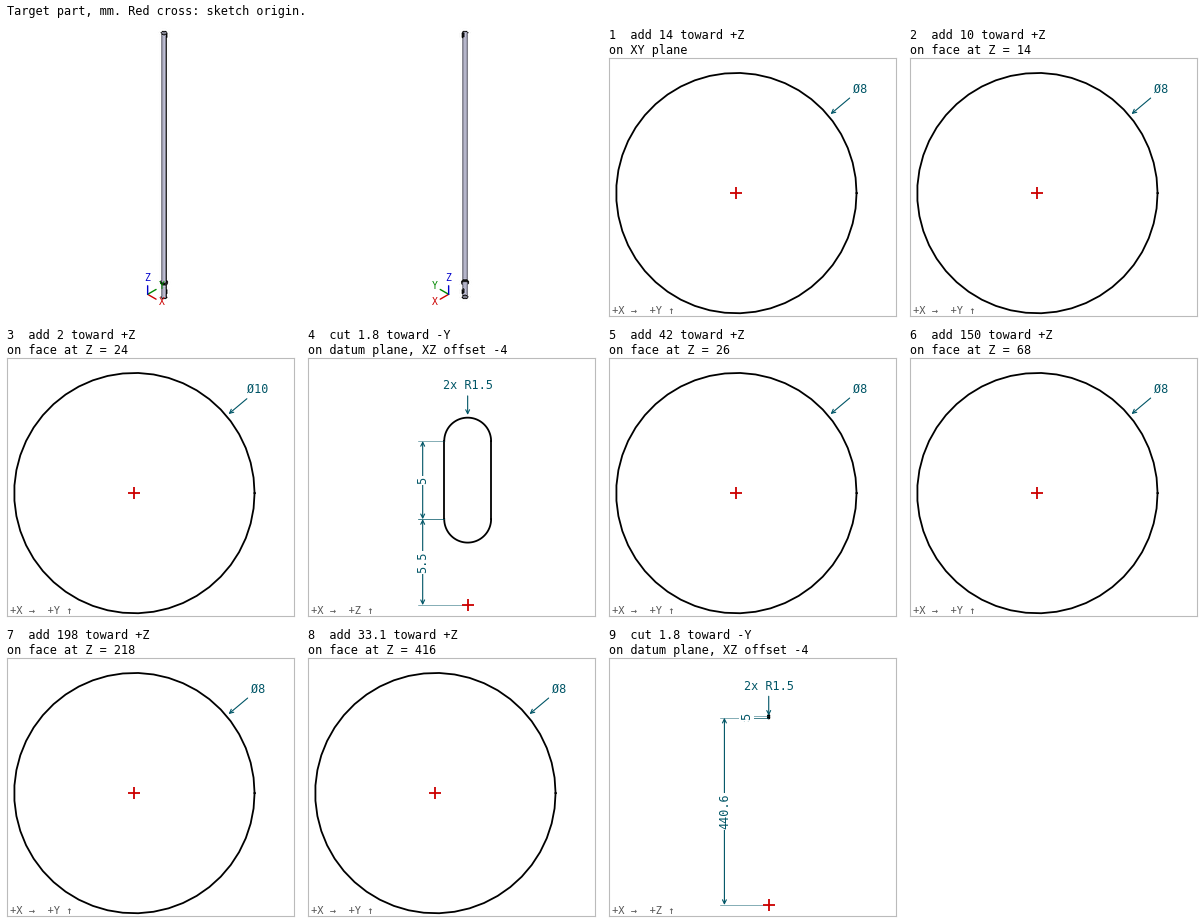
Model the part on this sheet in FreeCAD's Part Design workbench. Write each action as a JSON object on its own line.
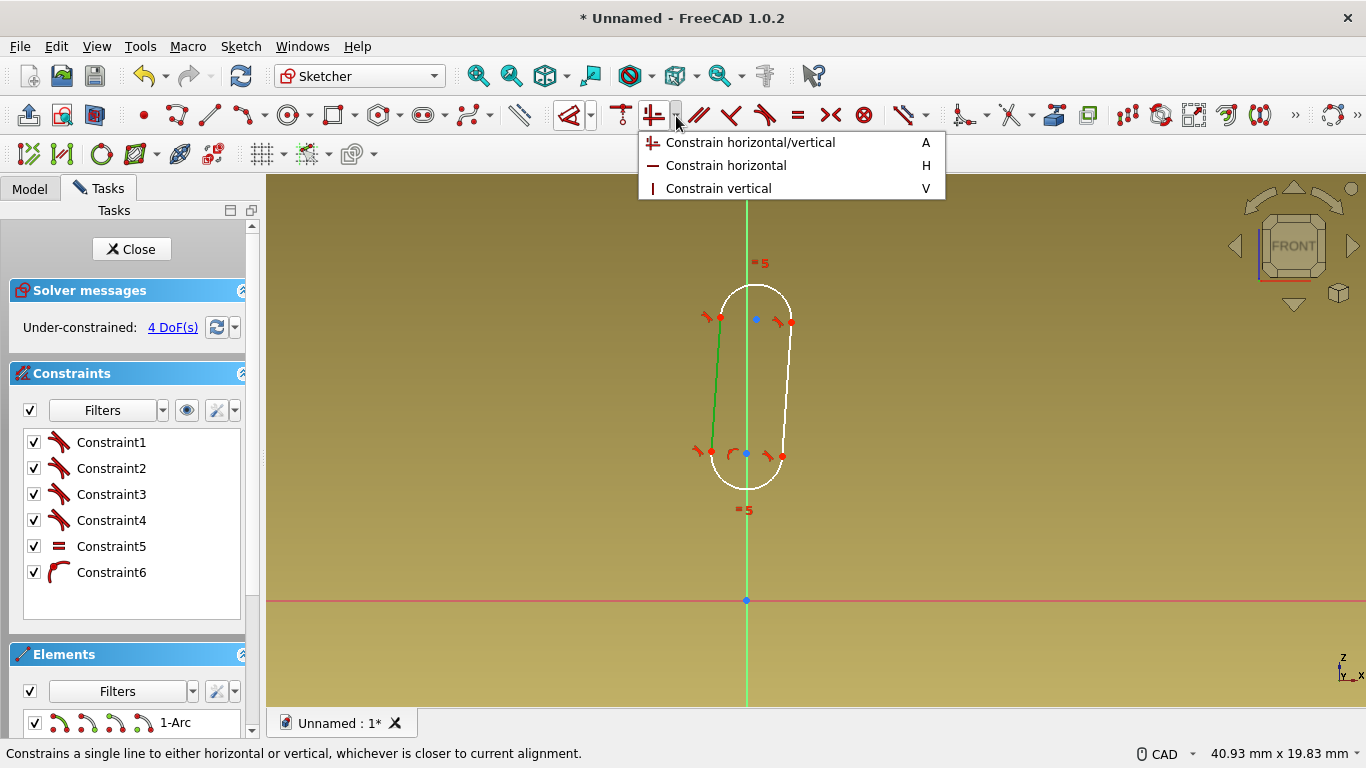
{"action": "left_click", "coordinate": [792, 188]}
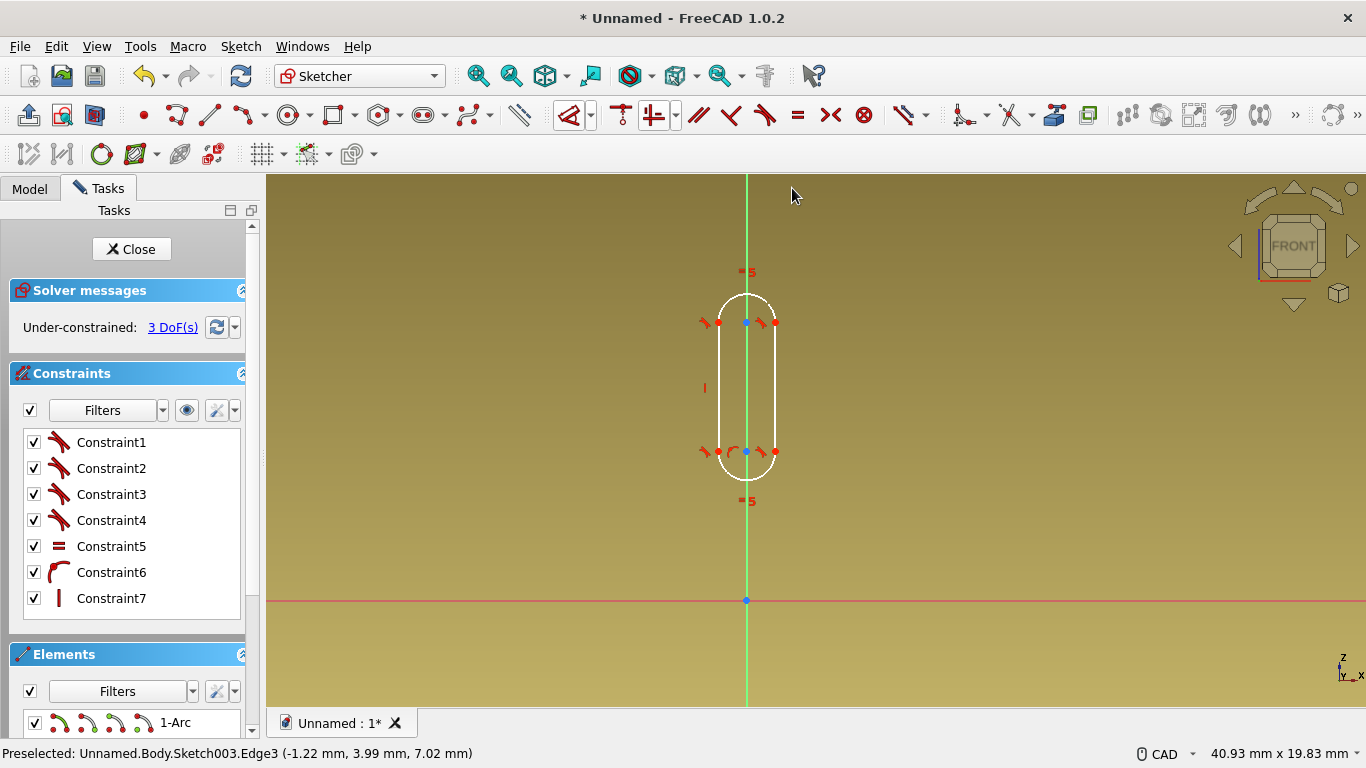
{"action": "left_click", "coordinate": [730, 475]}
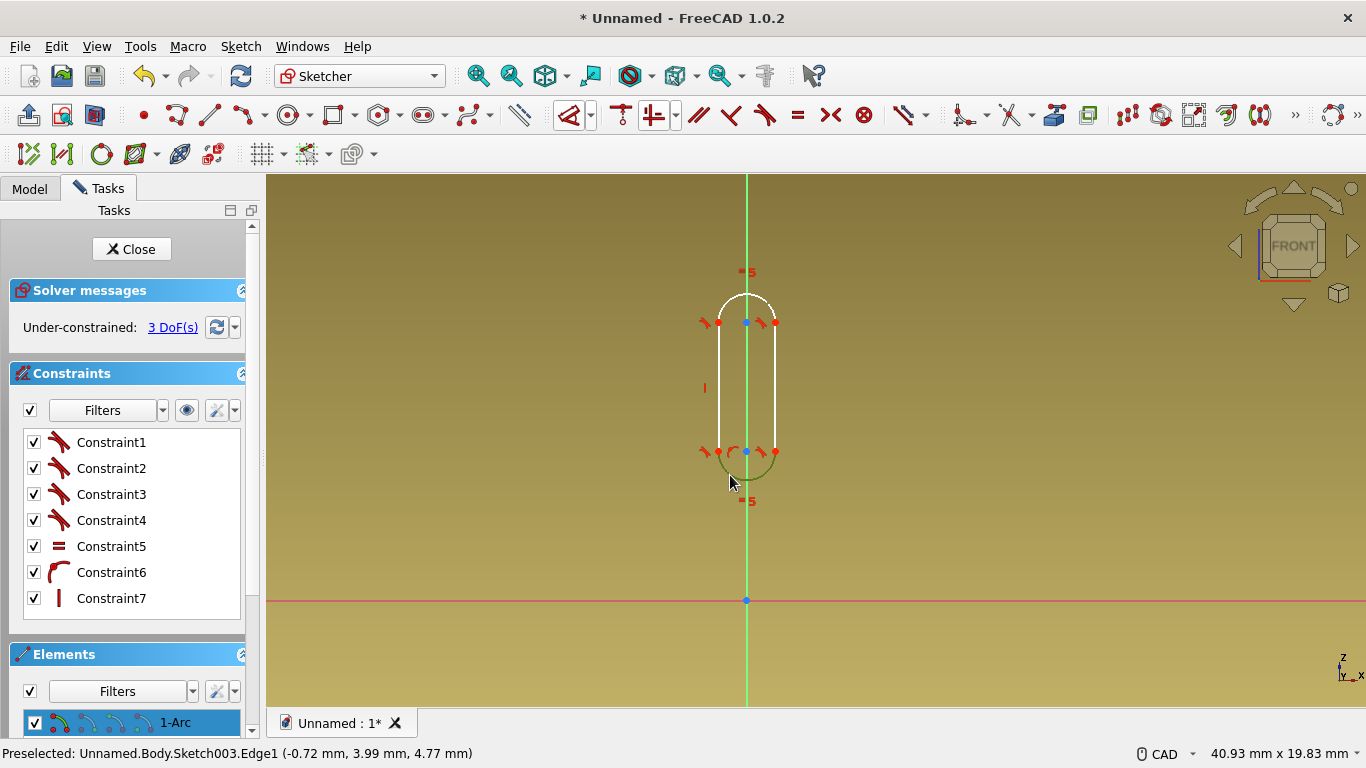
{"action": "left_click", "coordinate": [590, 116]}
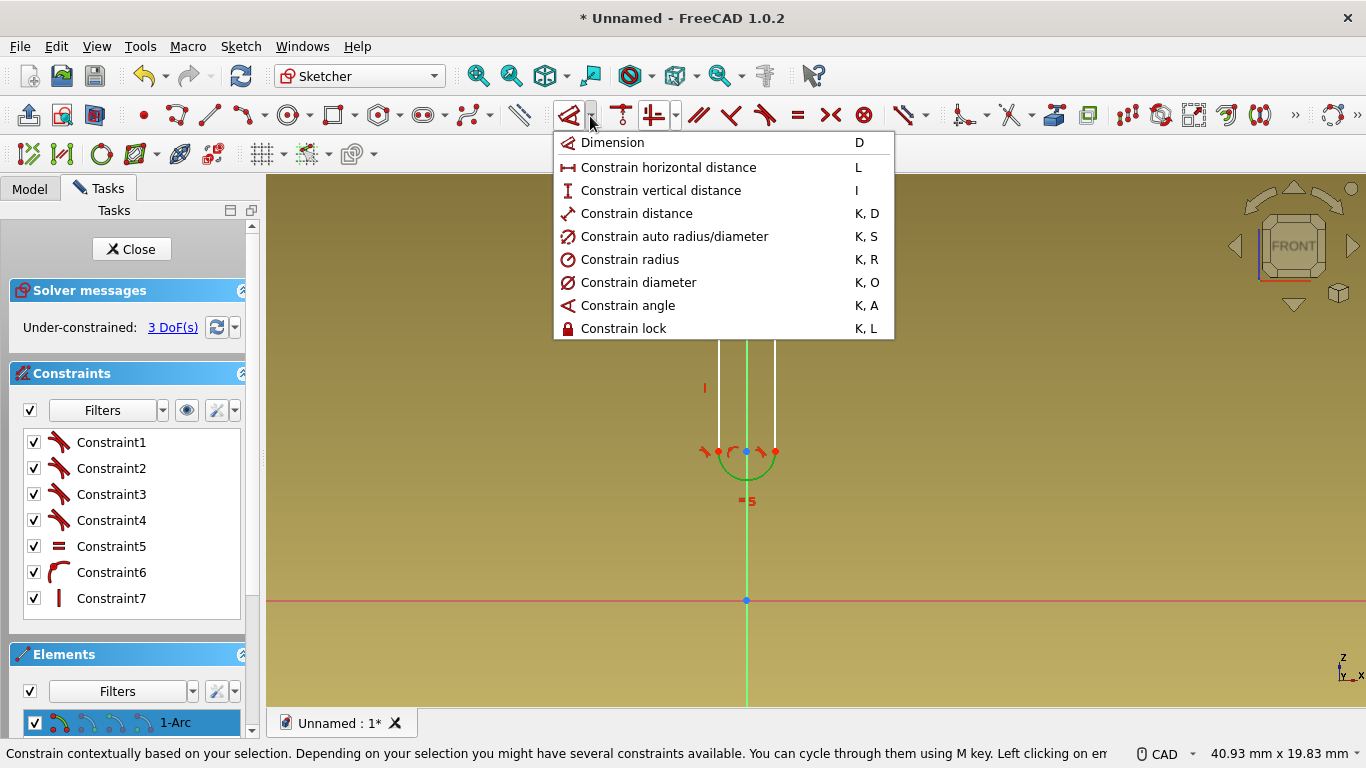
{"action": "left_click", "coordinate": [724, 260]}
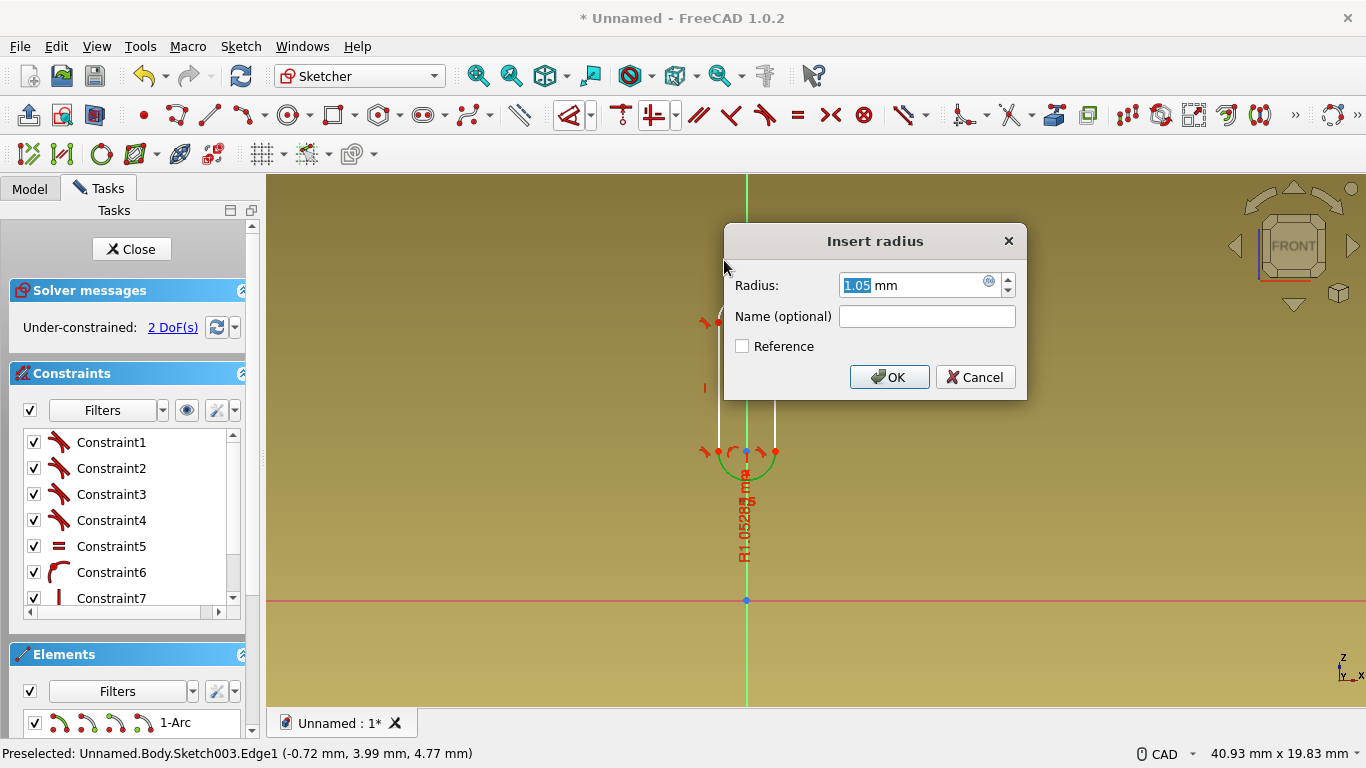
{"action": "type", "text": "1.5"}
{"action": "key", "text": "Return"}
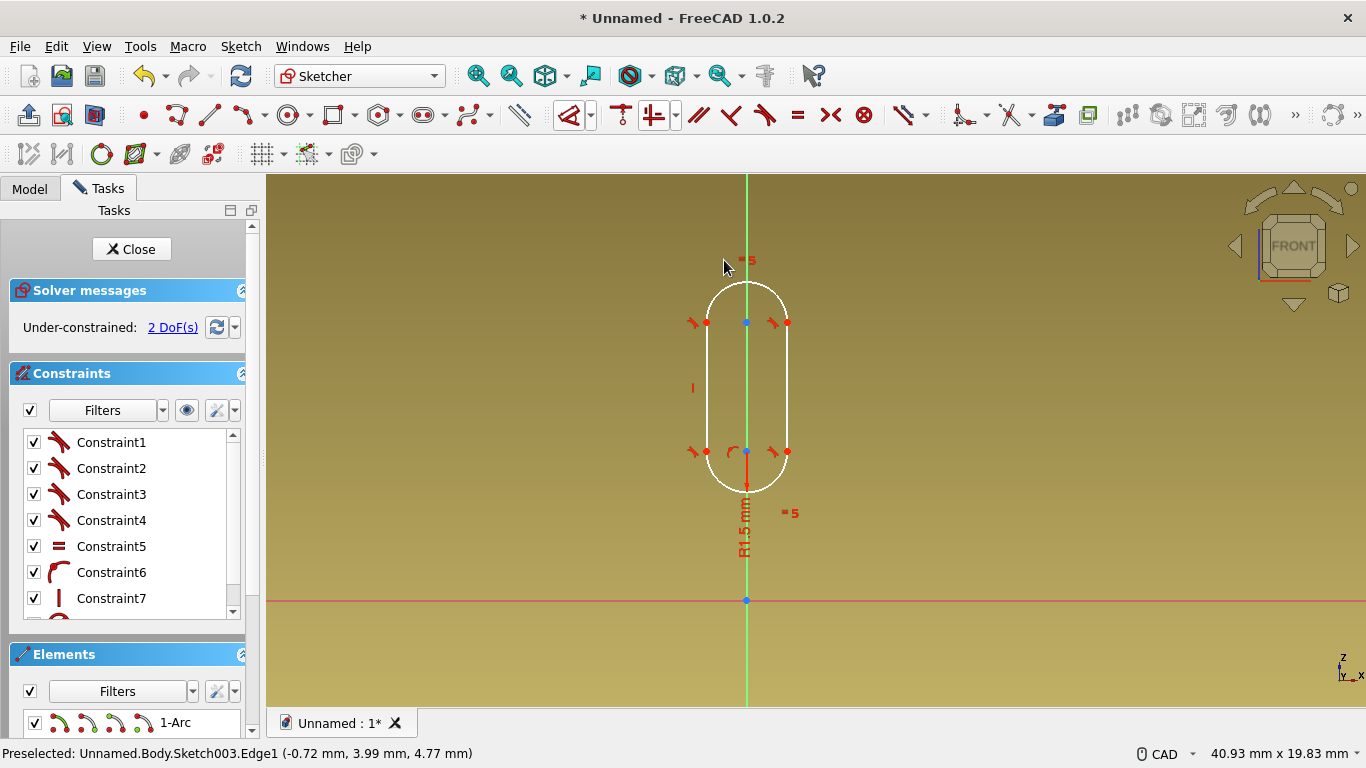
{"action": "left_click", "coordinate": [707, 413]}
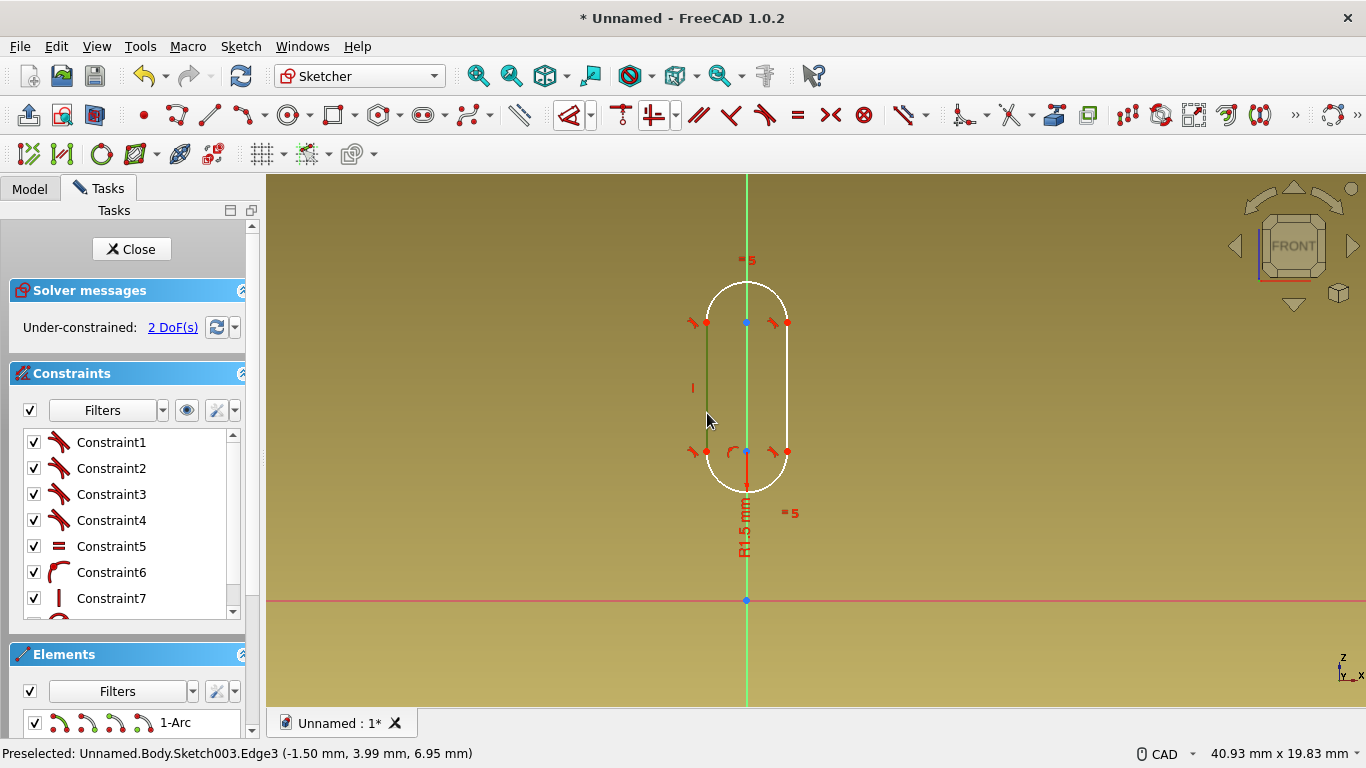
{"action": "key", "text": "i"}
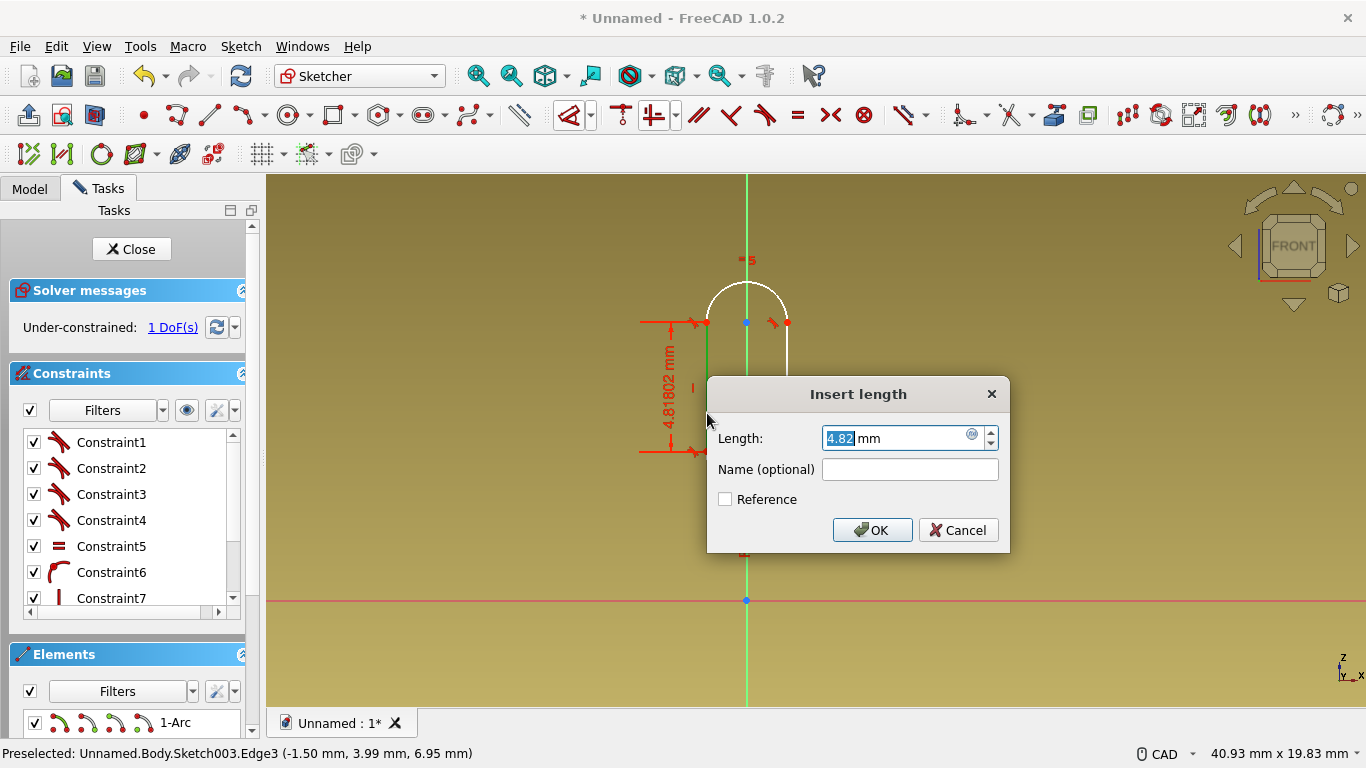
{"action": "type", "text": "5"}
{"action": "key", "text": "Return"}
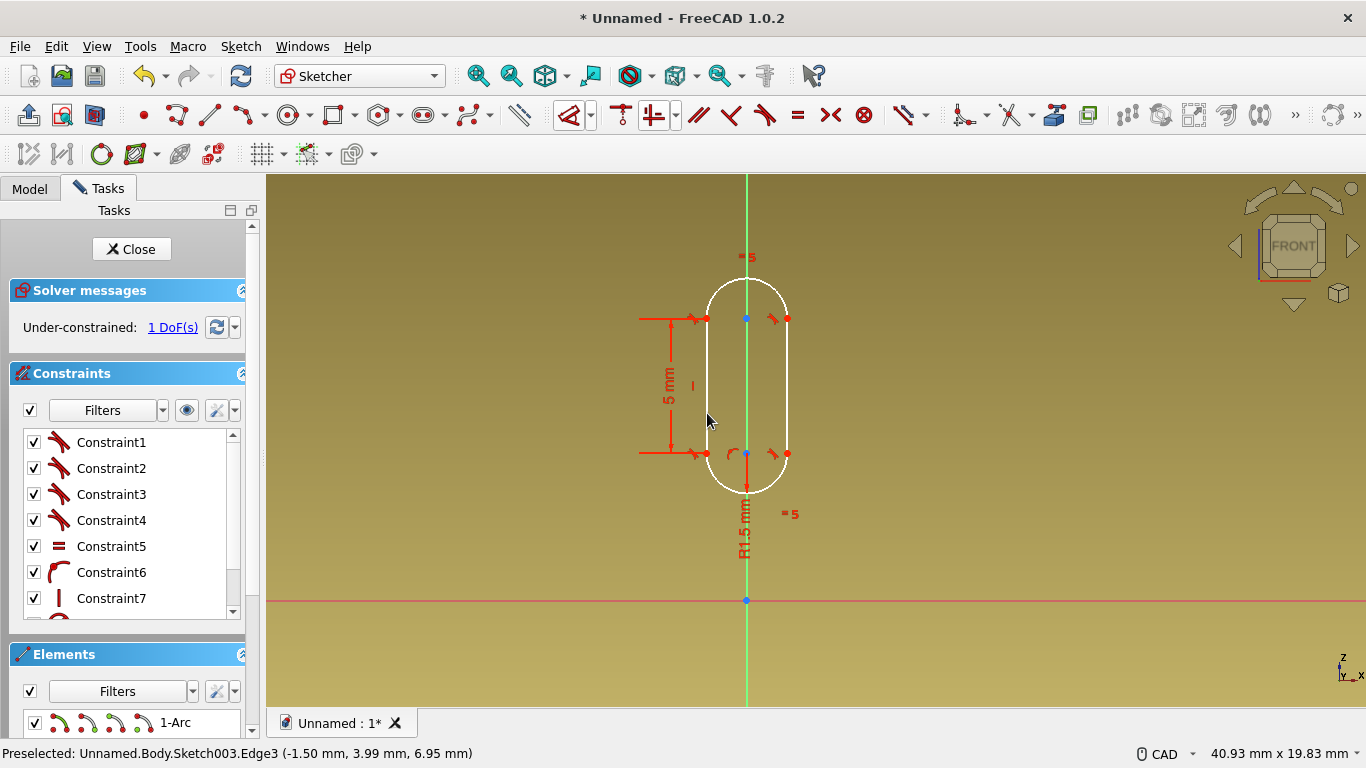
{"action": "left_click", "coordinate": [707, 453]}